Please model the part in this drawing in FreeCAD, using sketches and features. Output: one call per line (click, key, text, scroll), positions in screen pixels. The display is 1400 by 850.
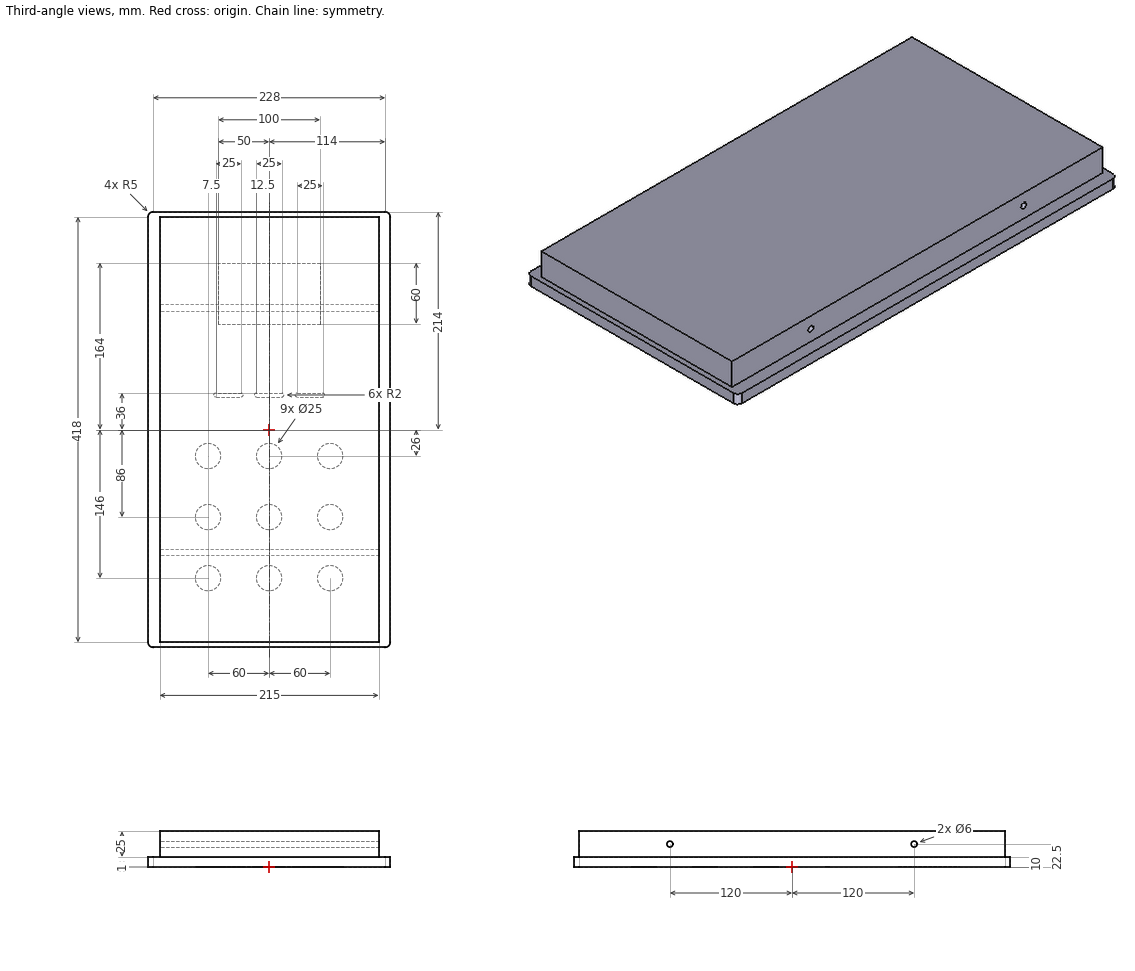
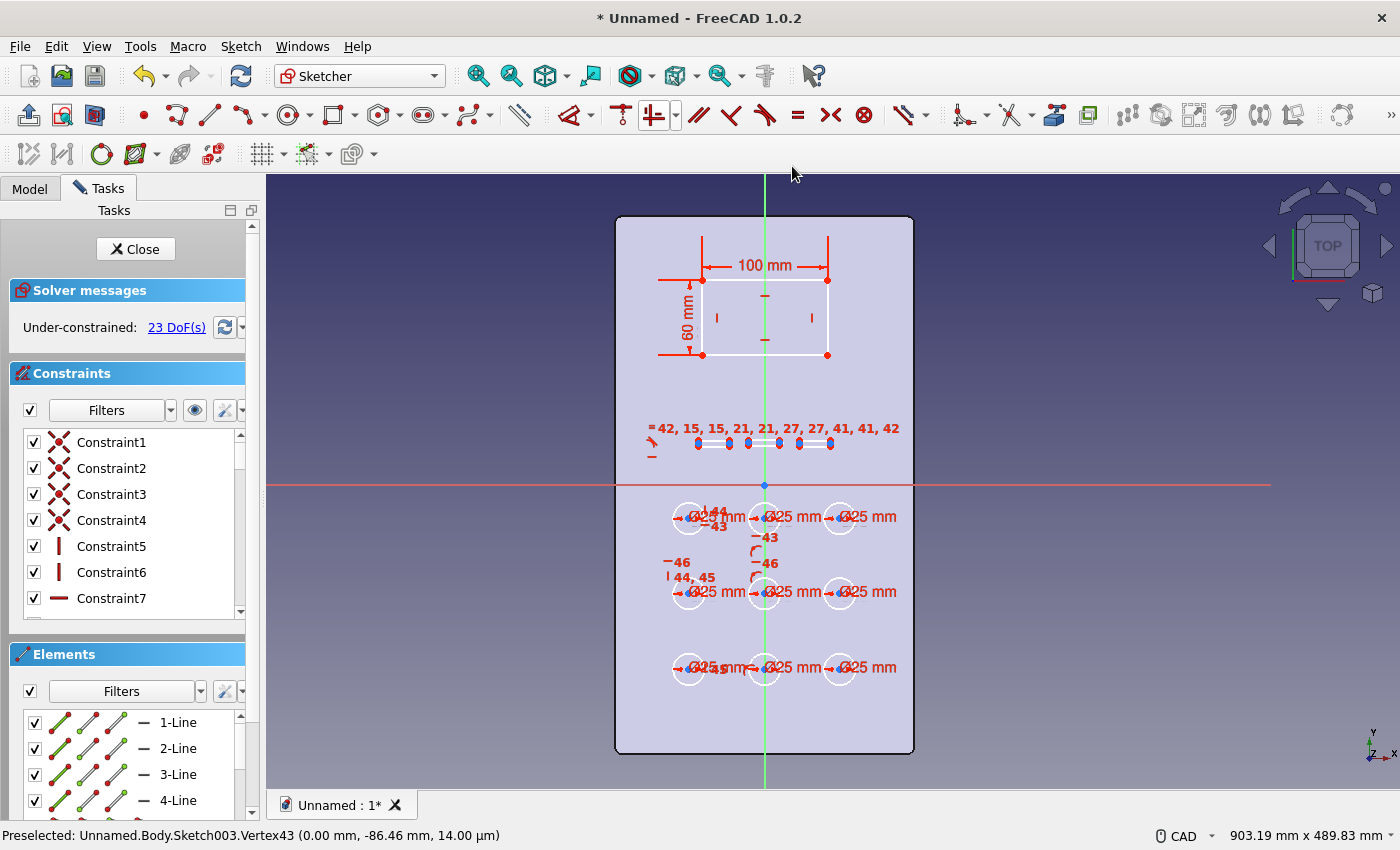
click(689, 669)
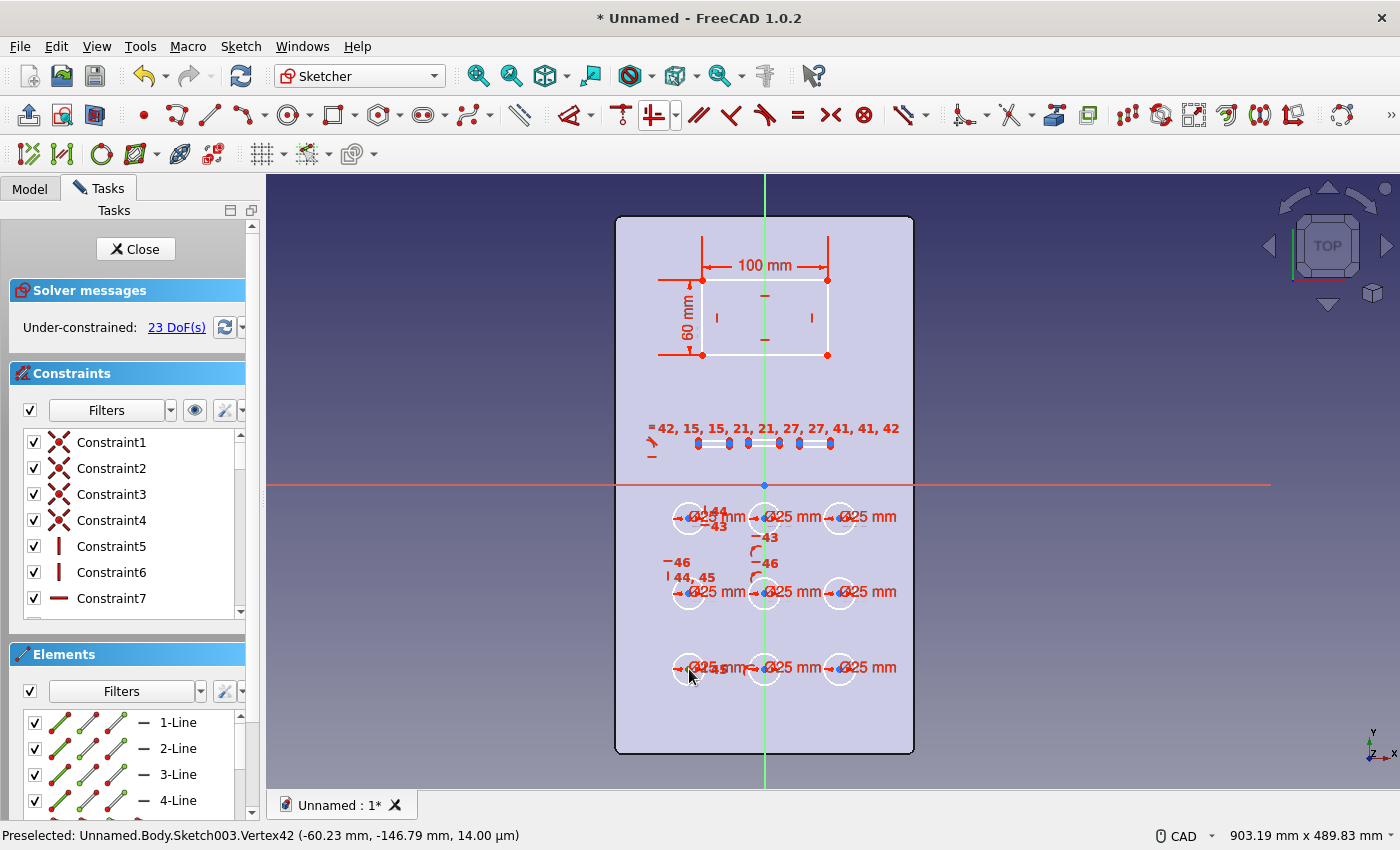
click(765, 669)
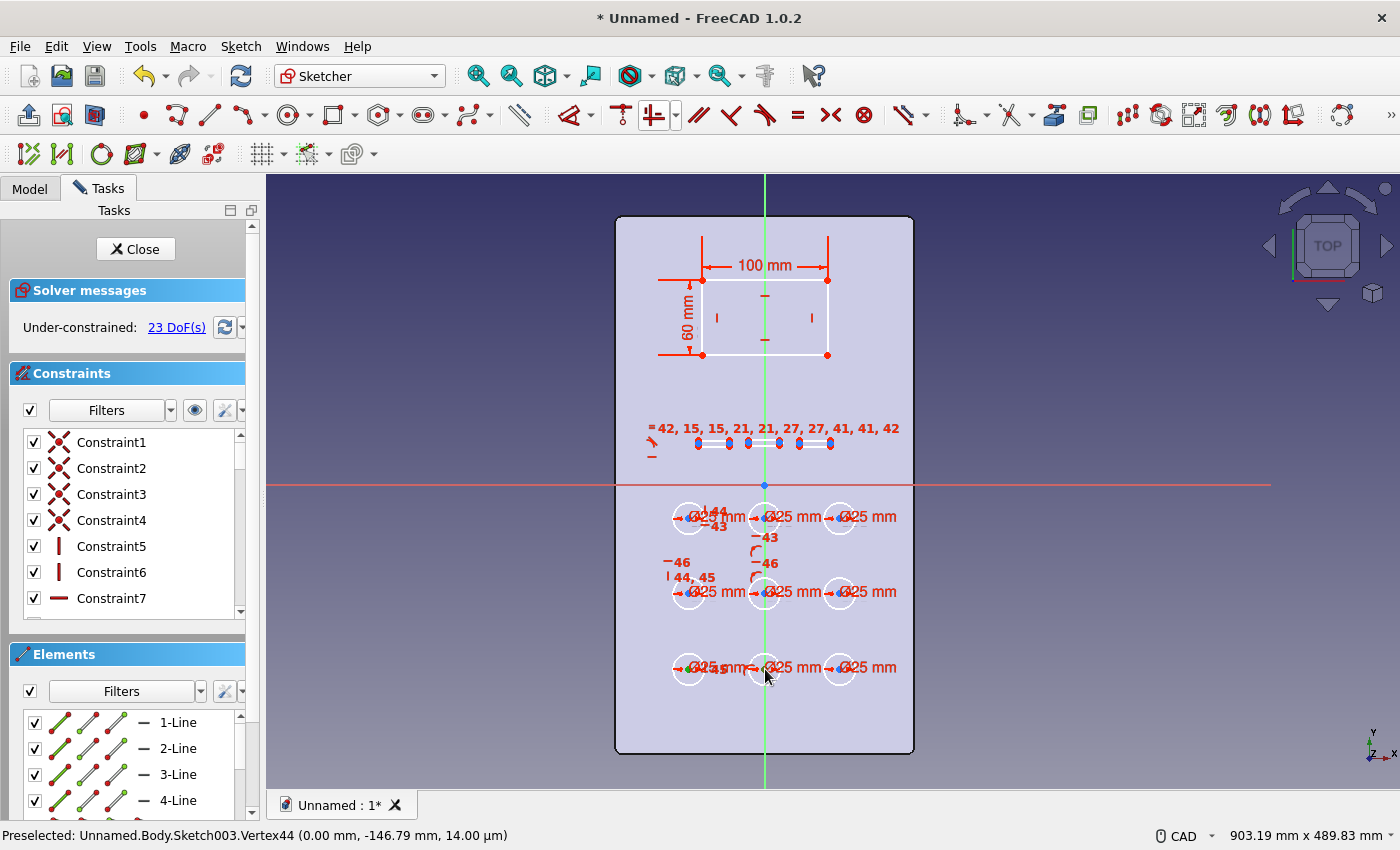
key(h)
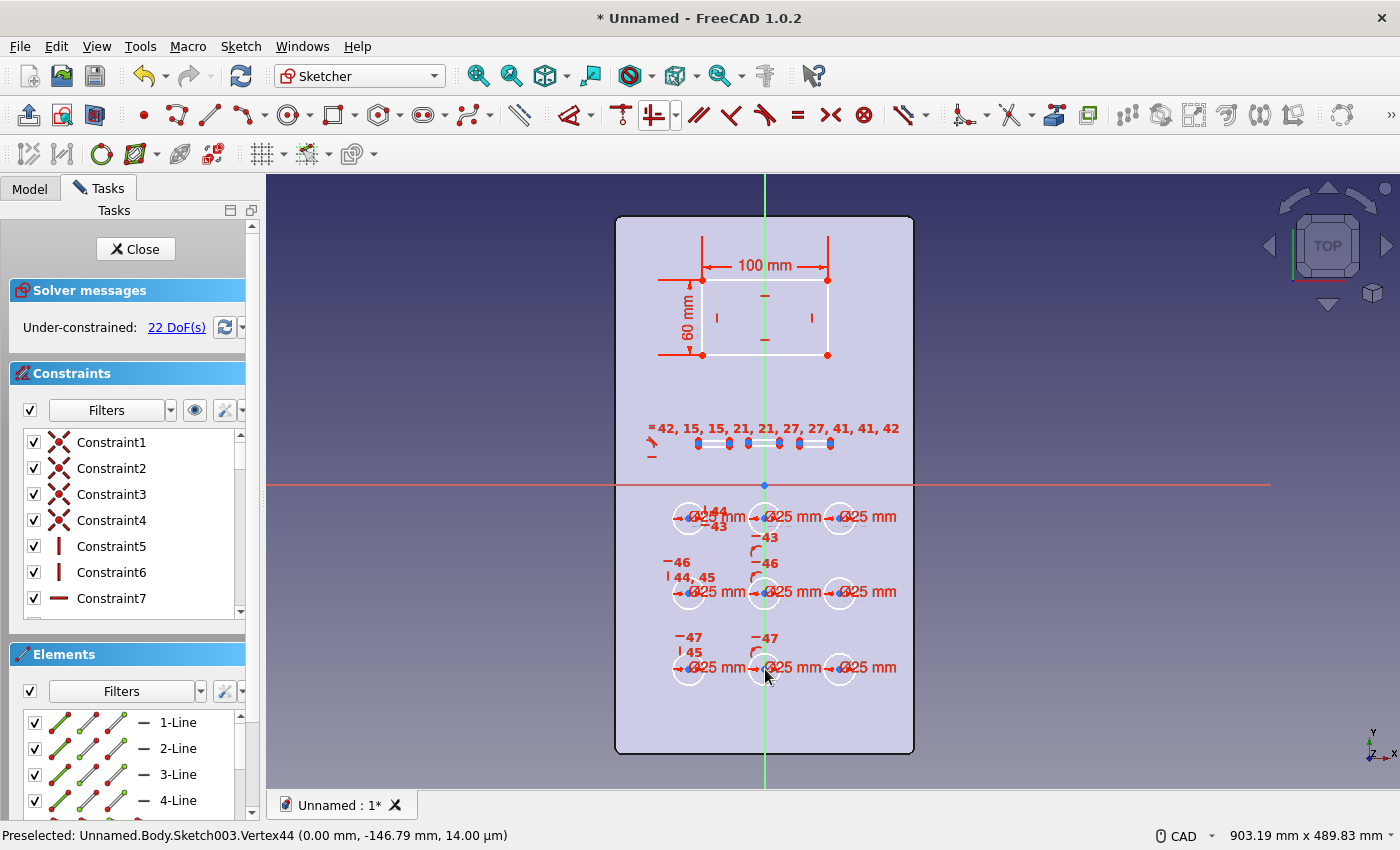
click(765, 669)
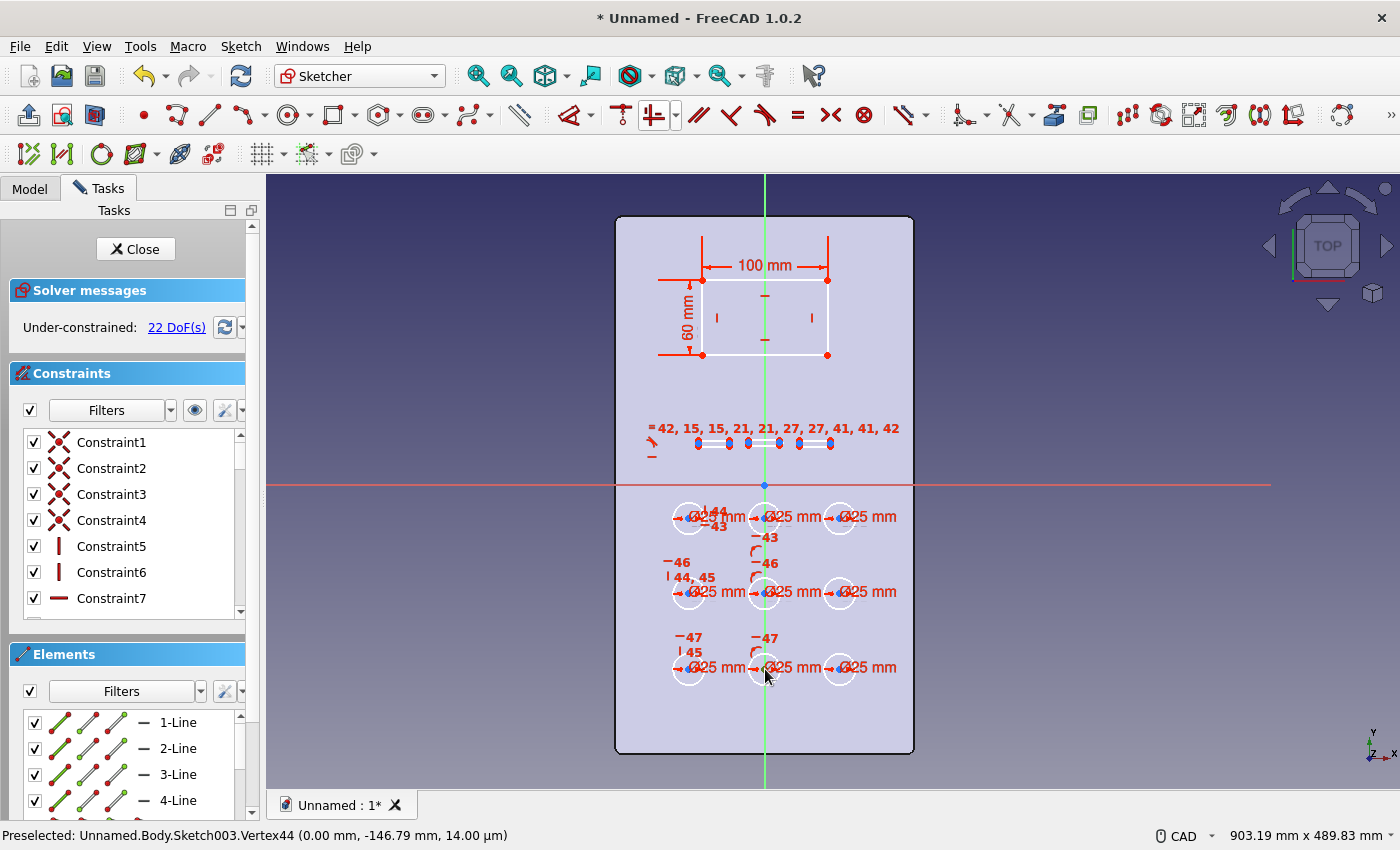
click(840, 669)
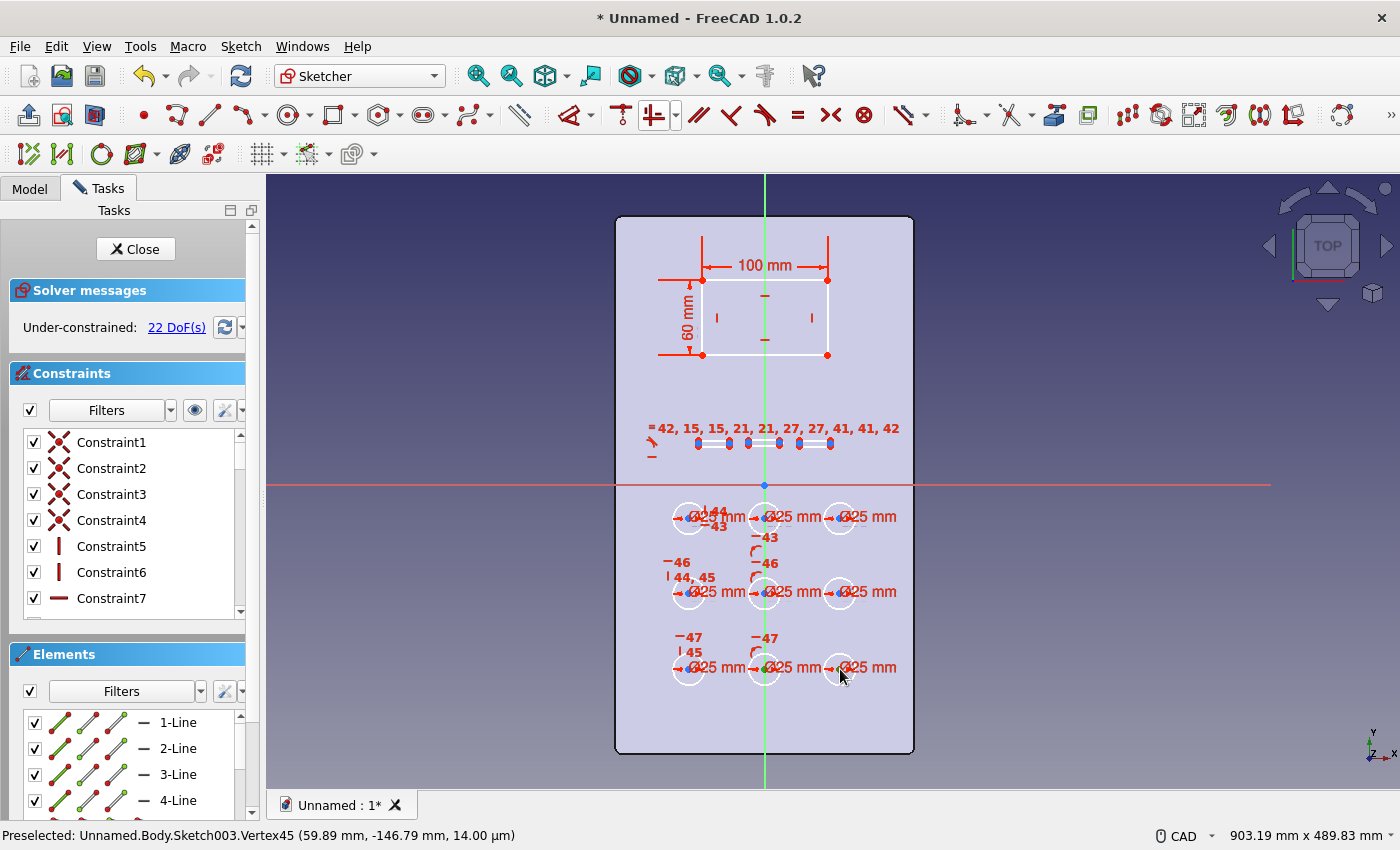
click(676, 116)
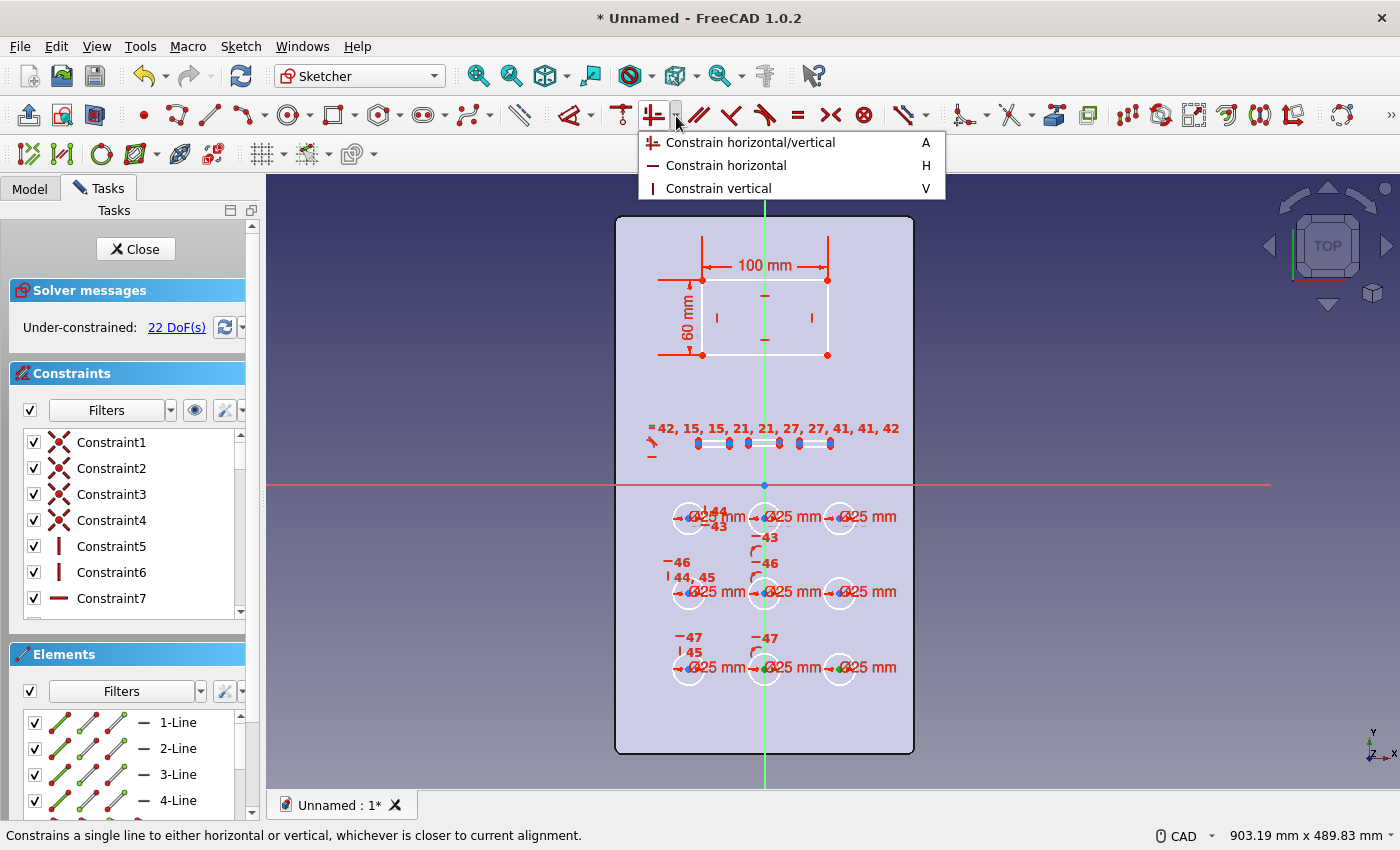
click(792, 166)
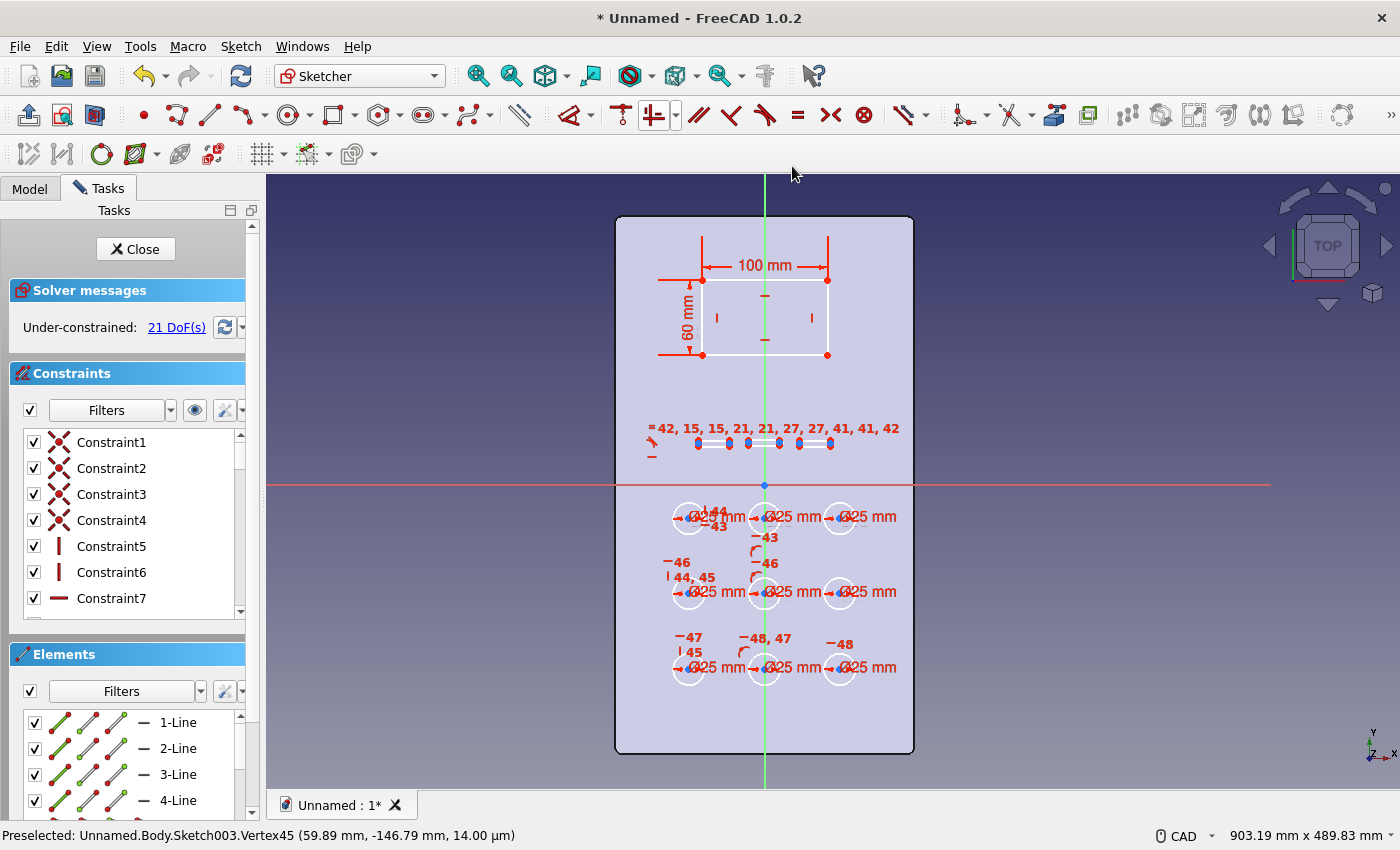
click(840, 669)